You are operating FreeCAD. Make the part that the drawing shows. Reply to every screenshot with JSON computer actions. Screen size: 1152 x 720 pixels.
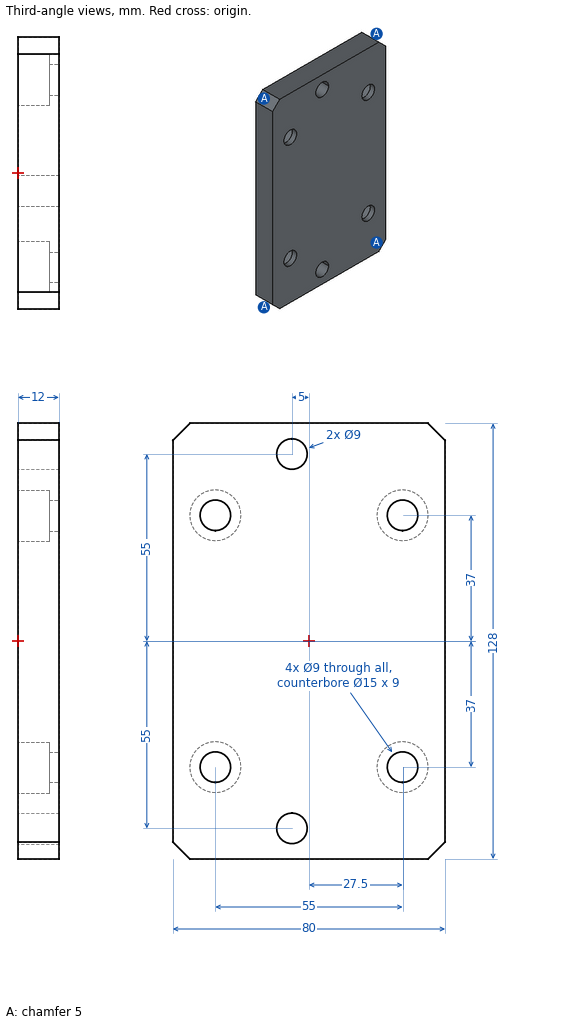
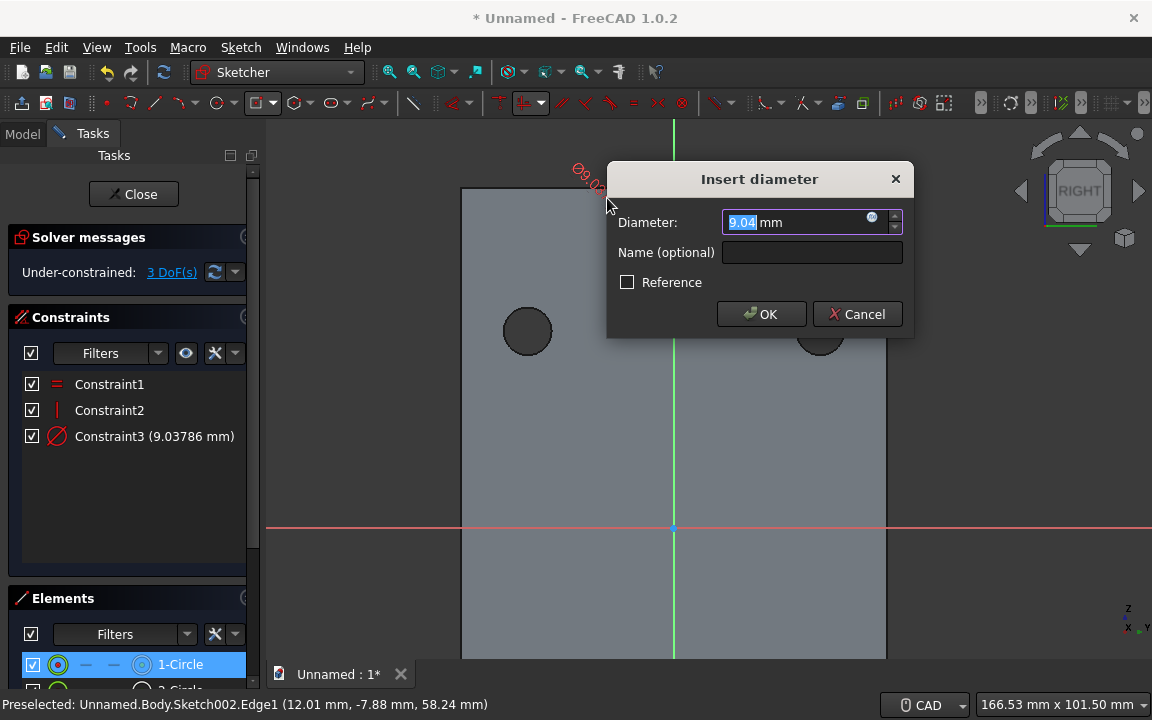
{"action": "type", "text": "9"}
{"action": "key", "text": "Return"}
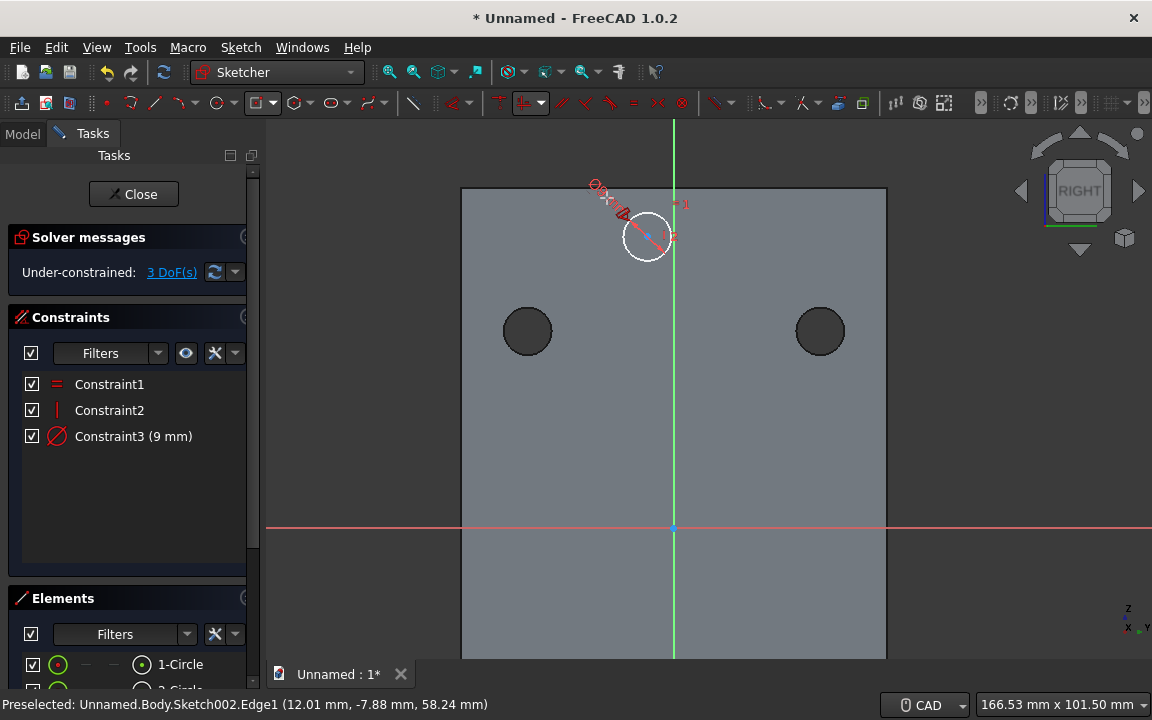
{"action": "scroll", "coordinate": [647, 237], "scroll_direction": "up", "scroll_amount": 3}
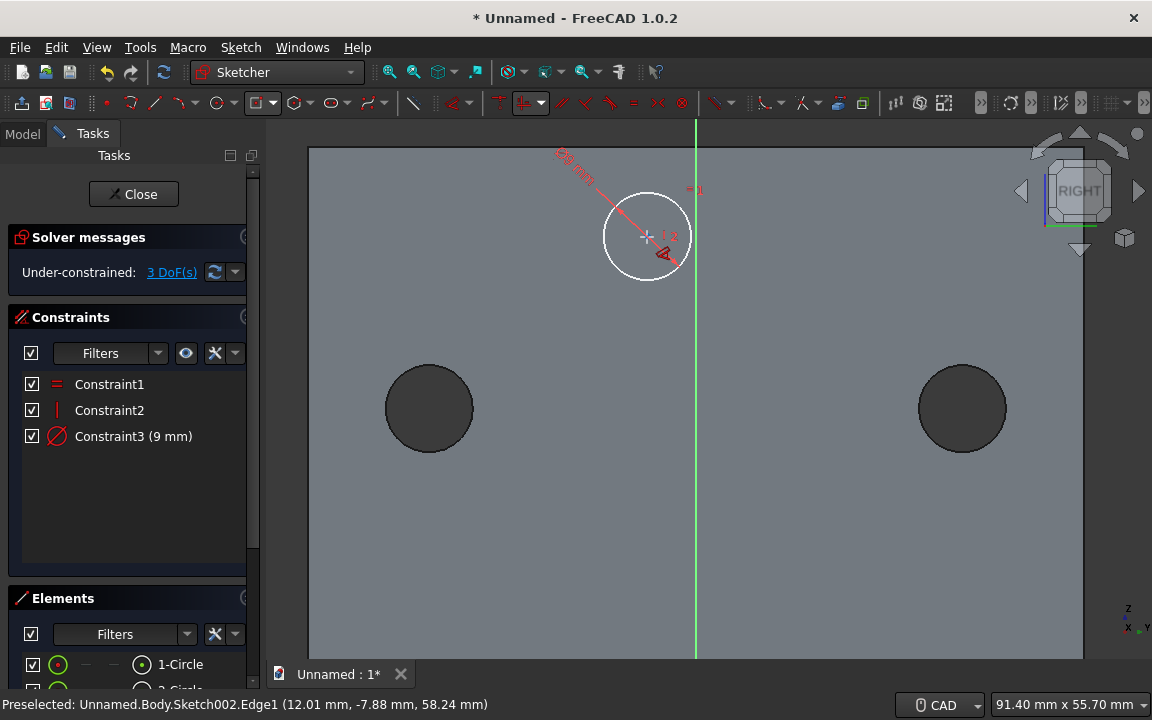
{"action": "left_click", "coordinate": [647, 237]}
{"action": "left_click", "coordinate": [672, 179]}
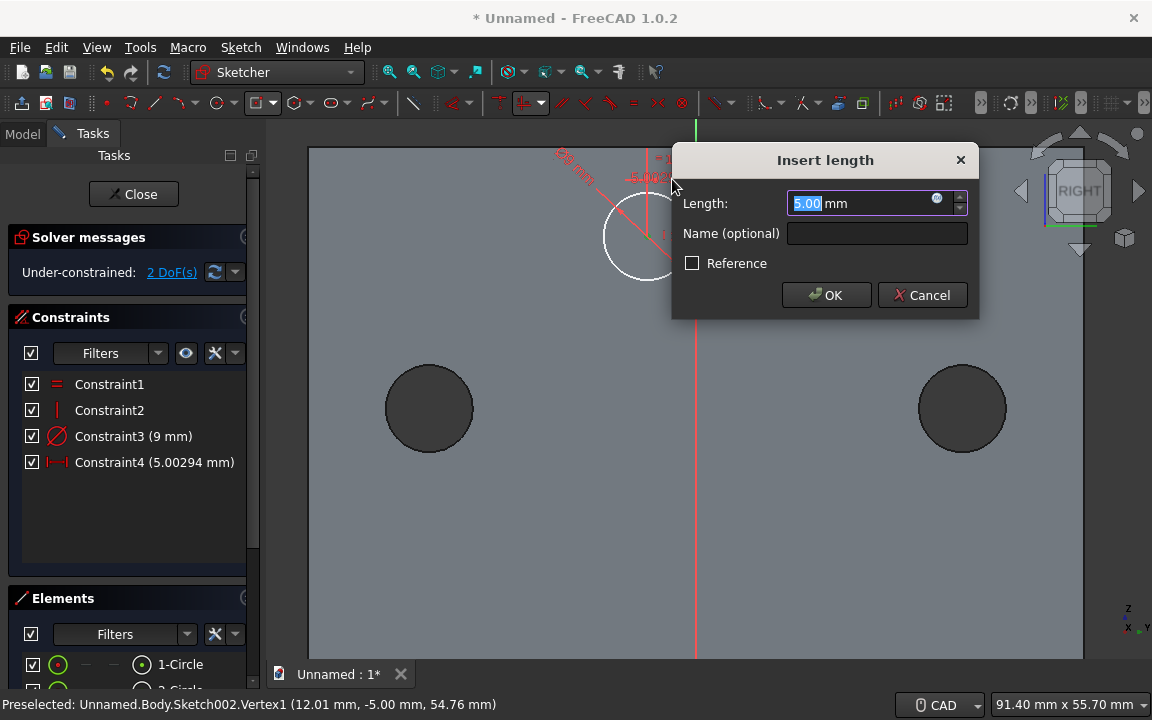
{"action": "type", "text": "5"}
{"action": "key", "text": "Return"}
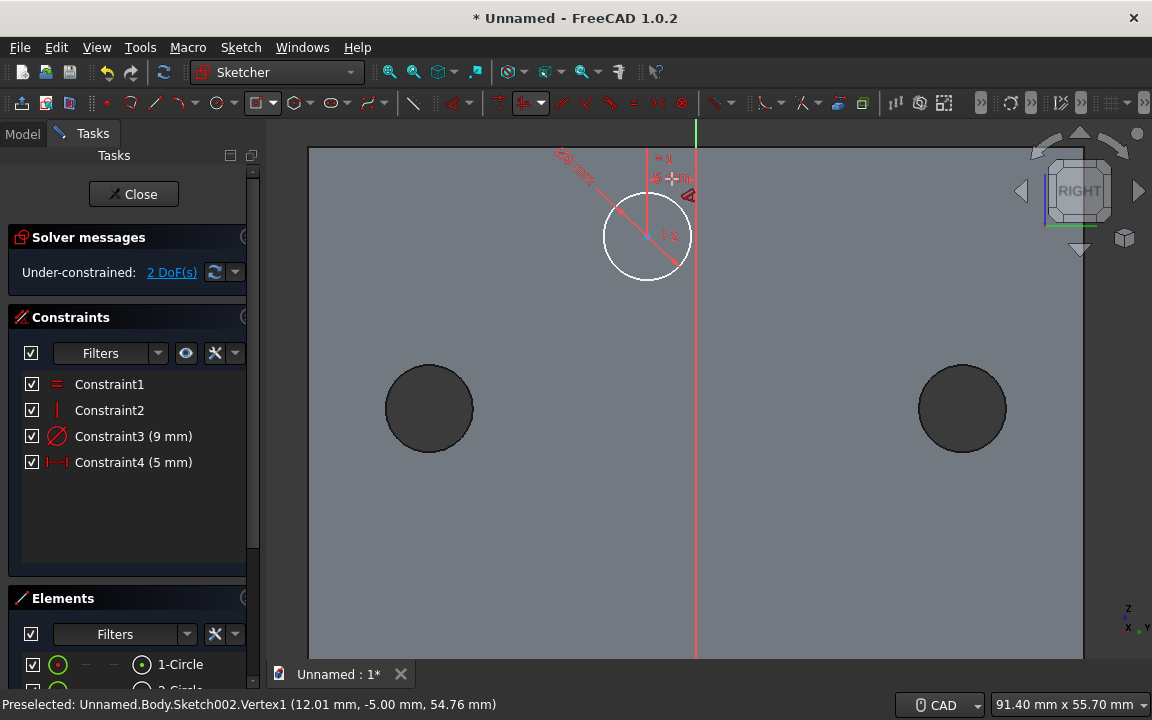
{"action": "left_click", "coordinate": [647, 237]}
{"action": "left_click", "coordinate": [730, 434]}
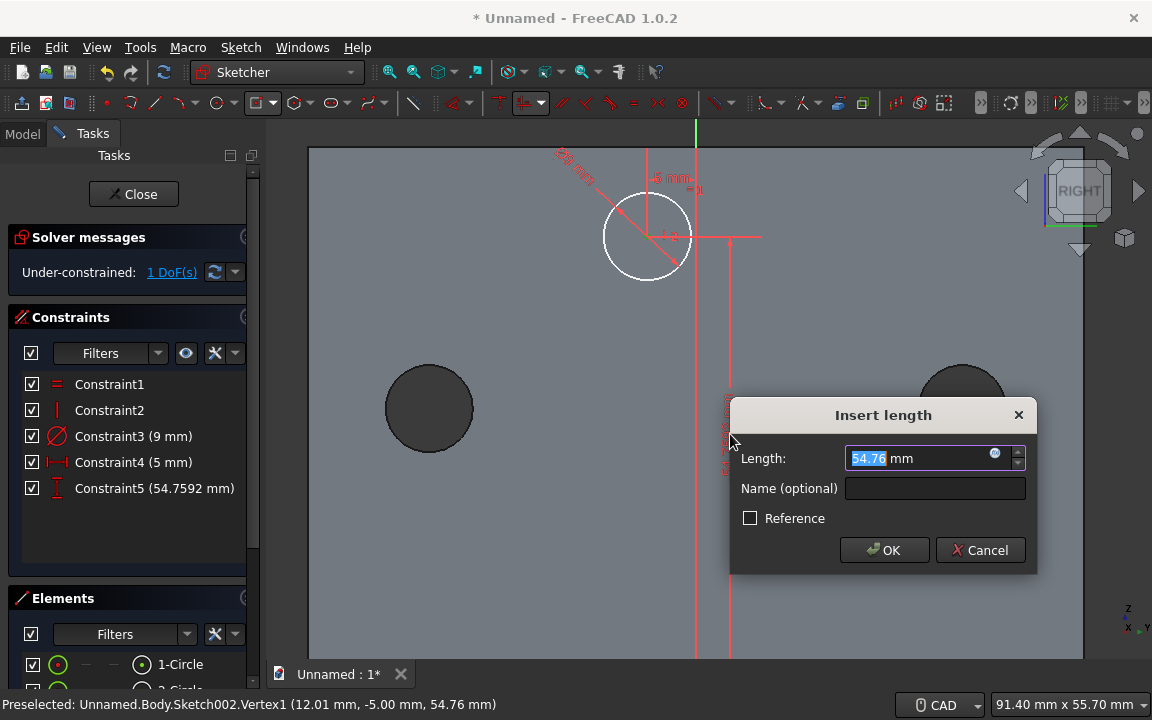
{"action": "type", "text": "55"}
{"action": "key", "text": "Return"}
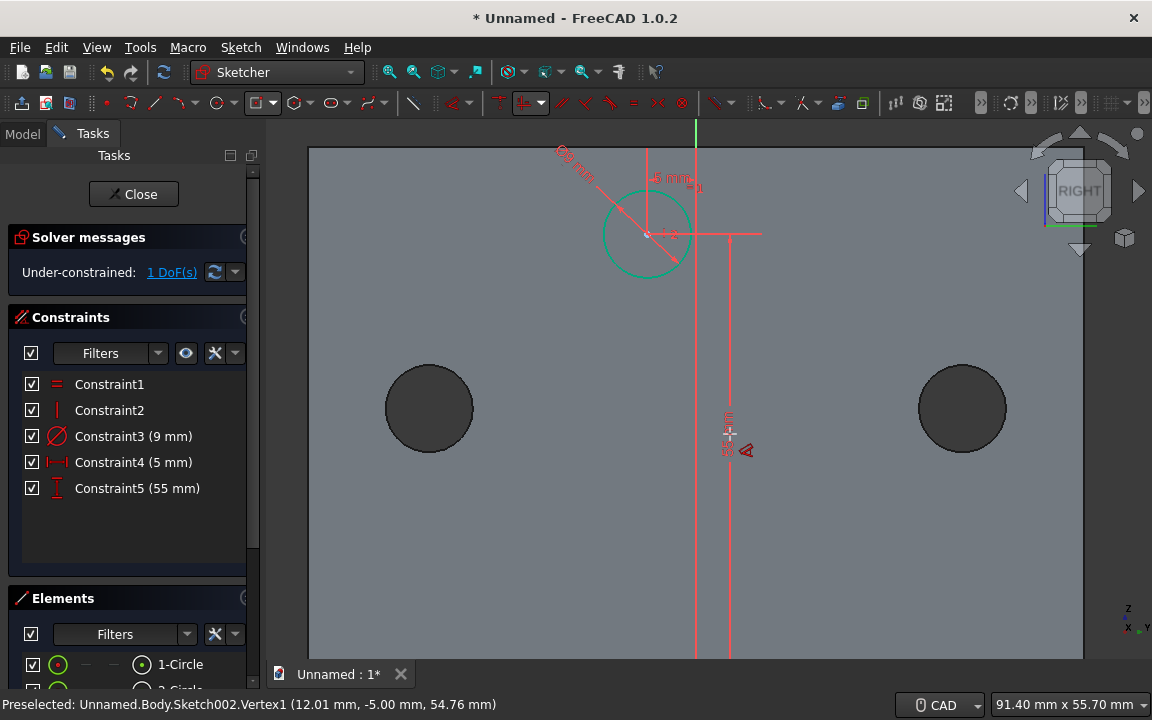
{"action": "scroll", "coordinate": [636, 226], "scroll_direction": "down", "scroll_amount": 6}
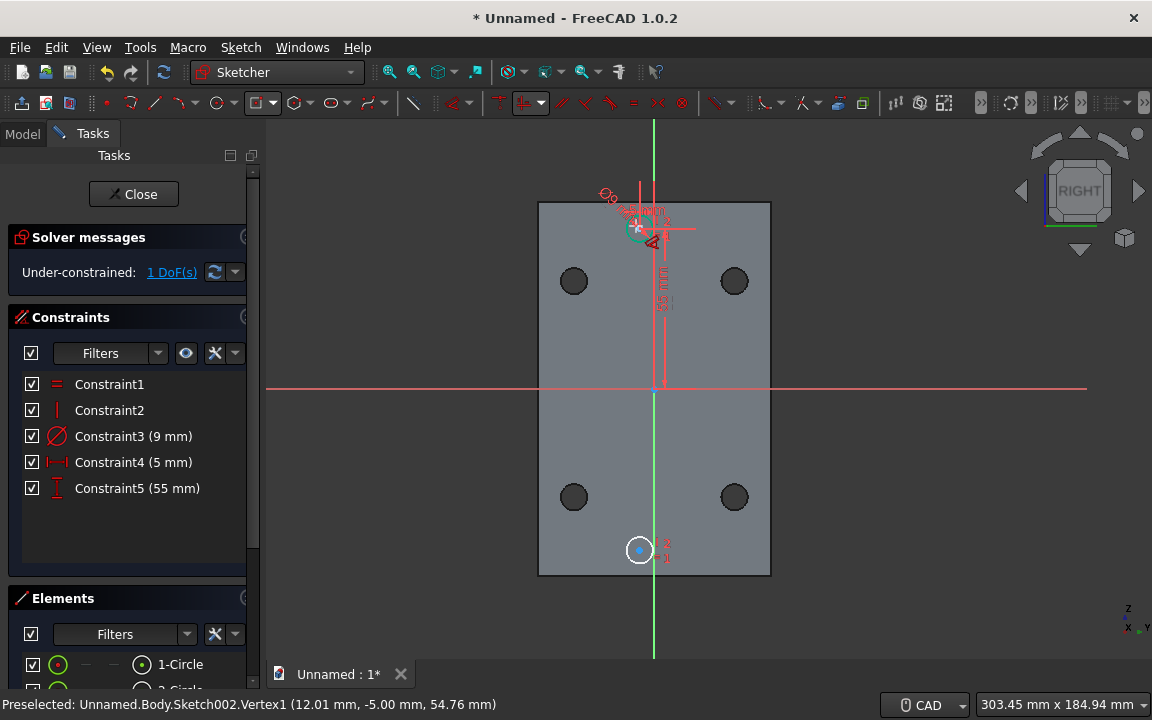
{"action": "left_click", "coordinate": [640, 550]}
{"action": "left_click", "coordinate": [688, 470]}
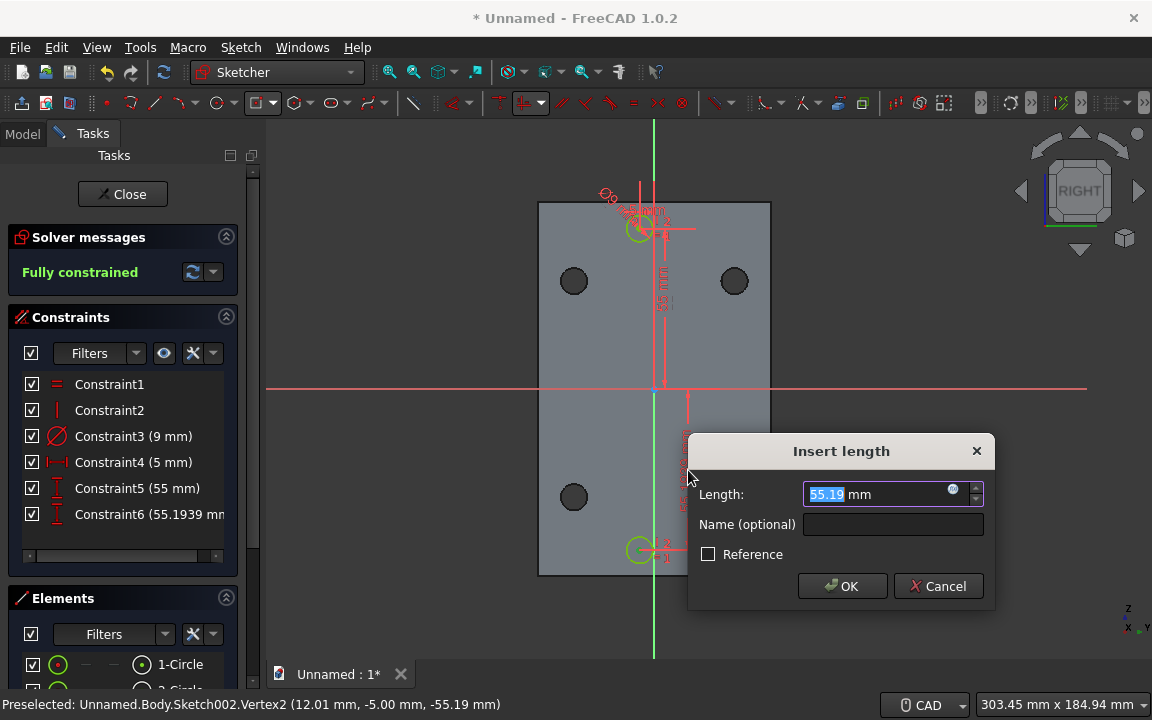
{"action": "type", "text": "55"}
{"action": "key", "text": "Return"}
{"action": "key", "text": "Escape"}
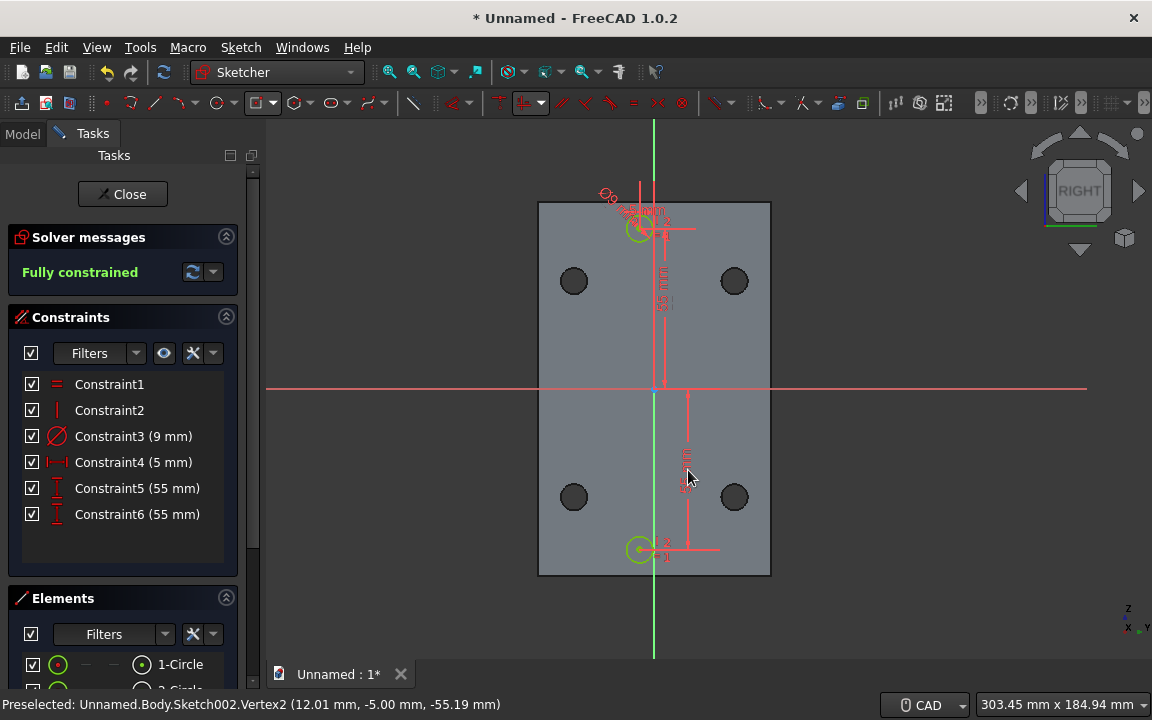
{"action": "left_click", "coordinate": [123, 194]}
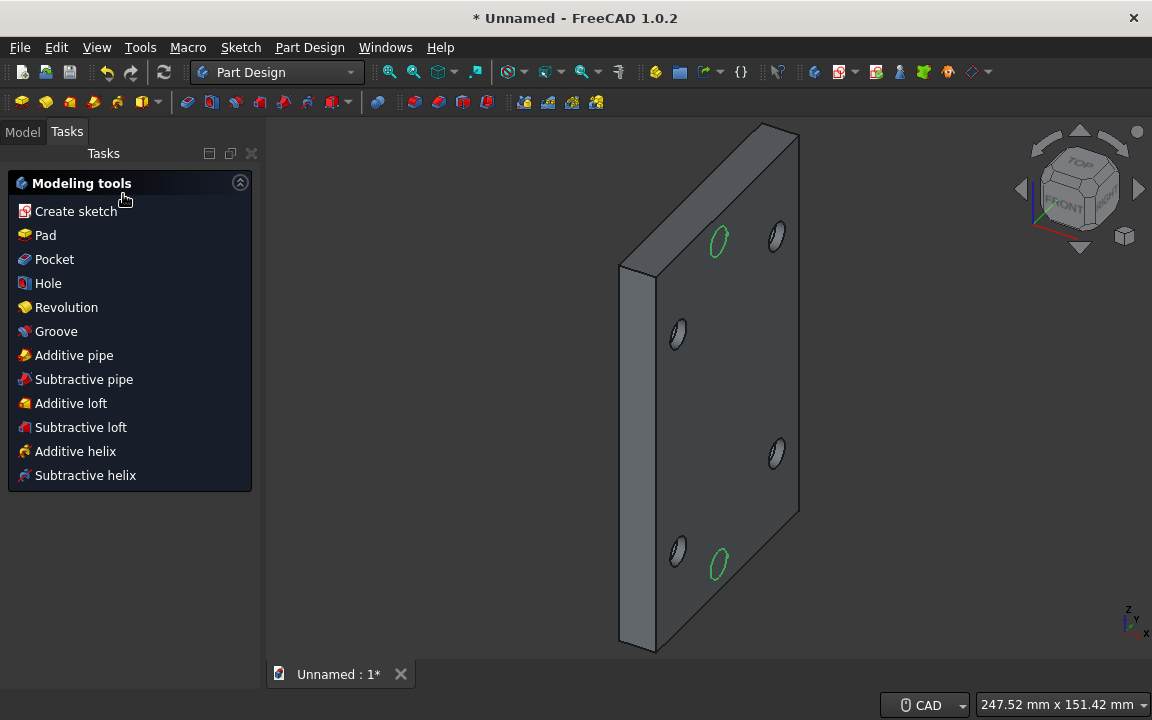
{"action": "left_click", "coordinate": [188, 102]}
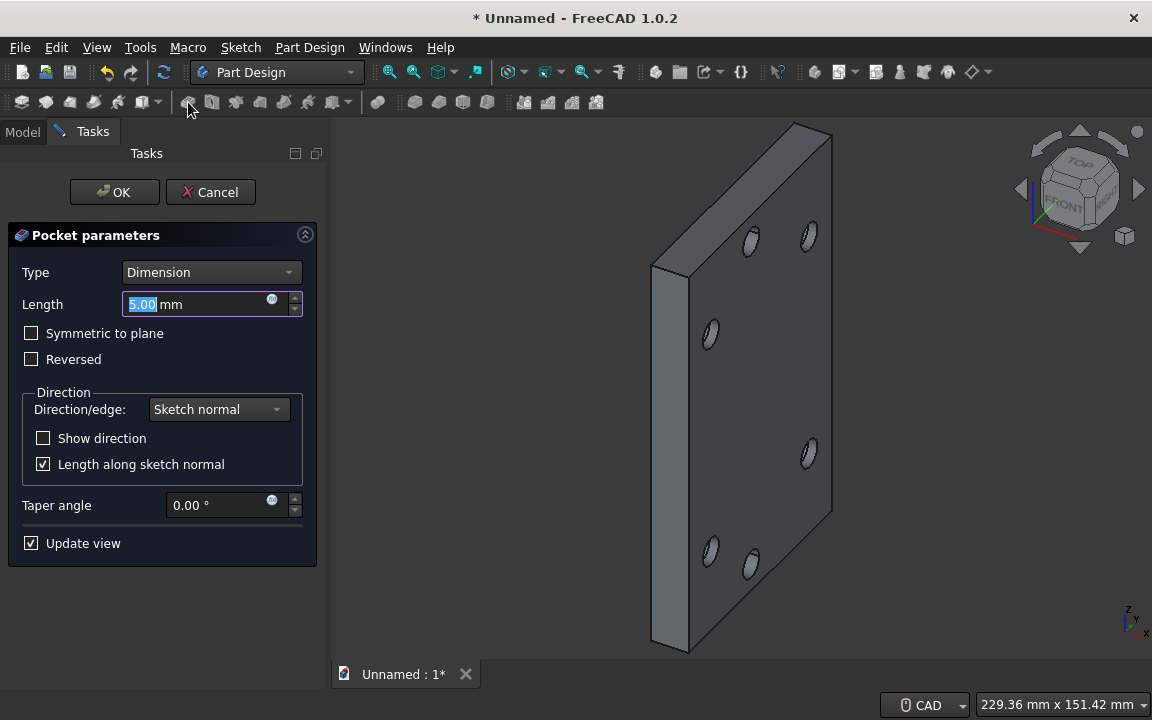
{"action": "left_click", "coordinate": [212, 272]}